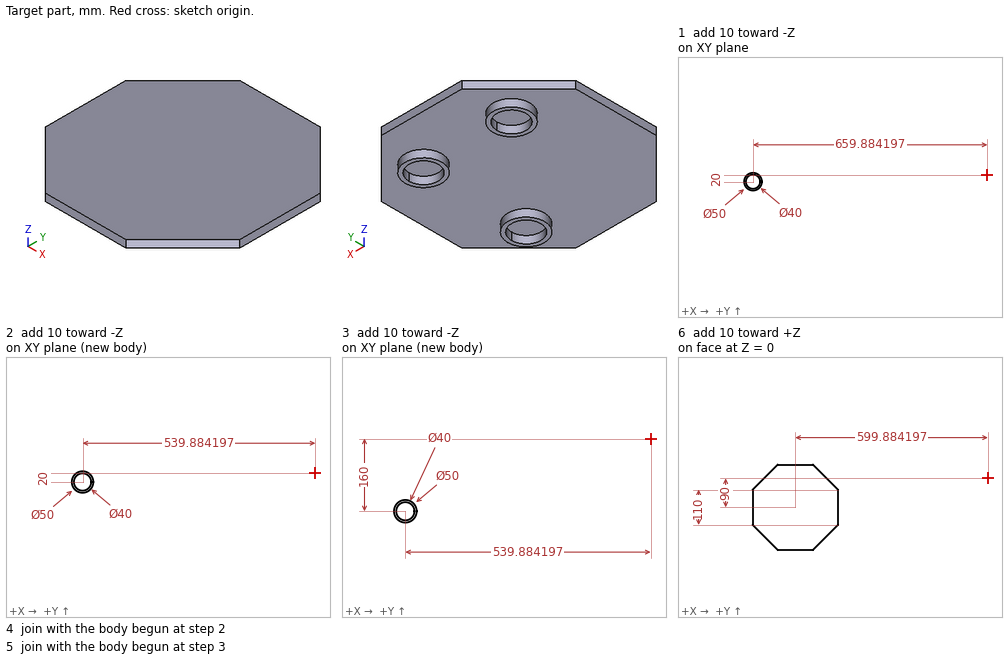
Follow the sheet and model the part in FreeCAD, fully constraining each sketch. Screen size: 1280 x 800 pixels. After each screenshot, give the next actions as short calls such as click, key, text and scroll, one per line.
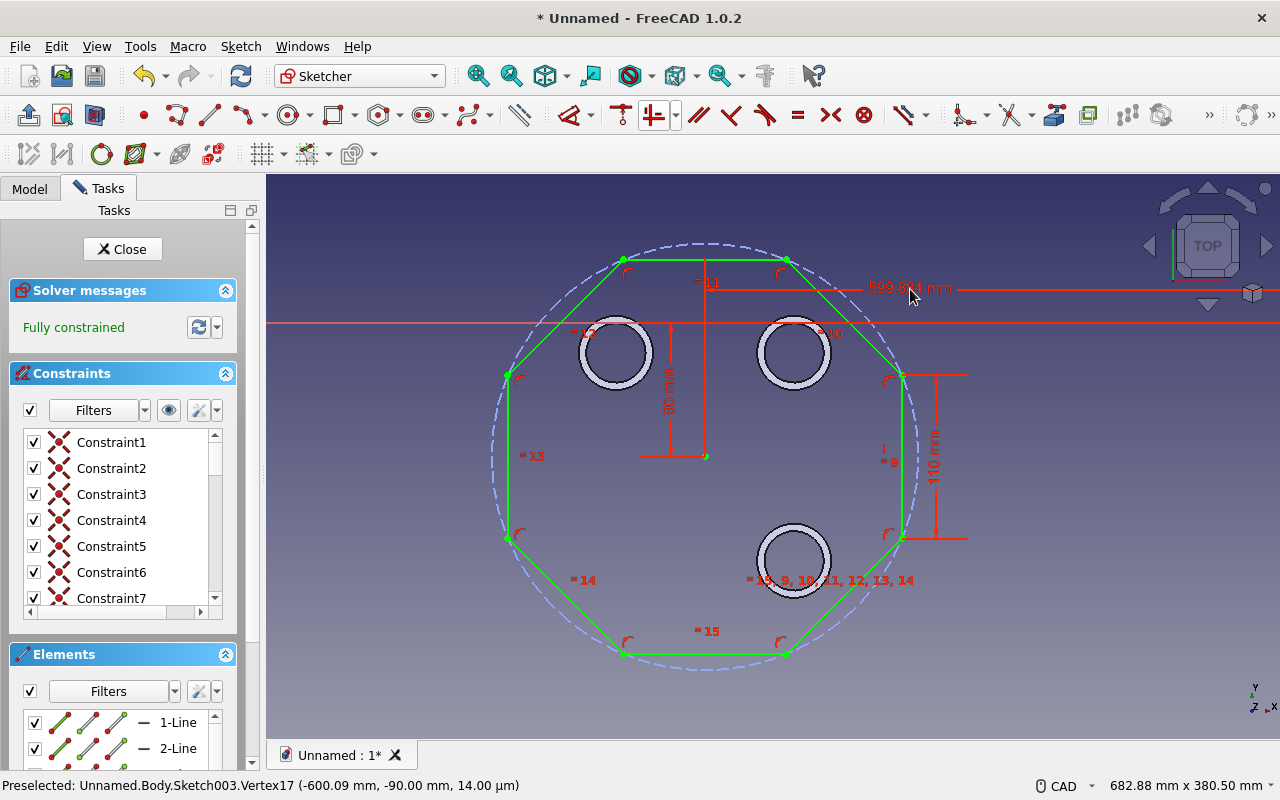
click(123, 249)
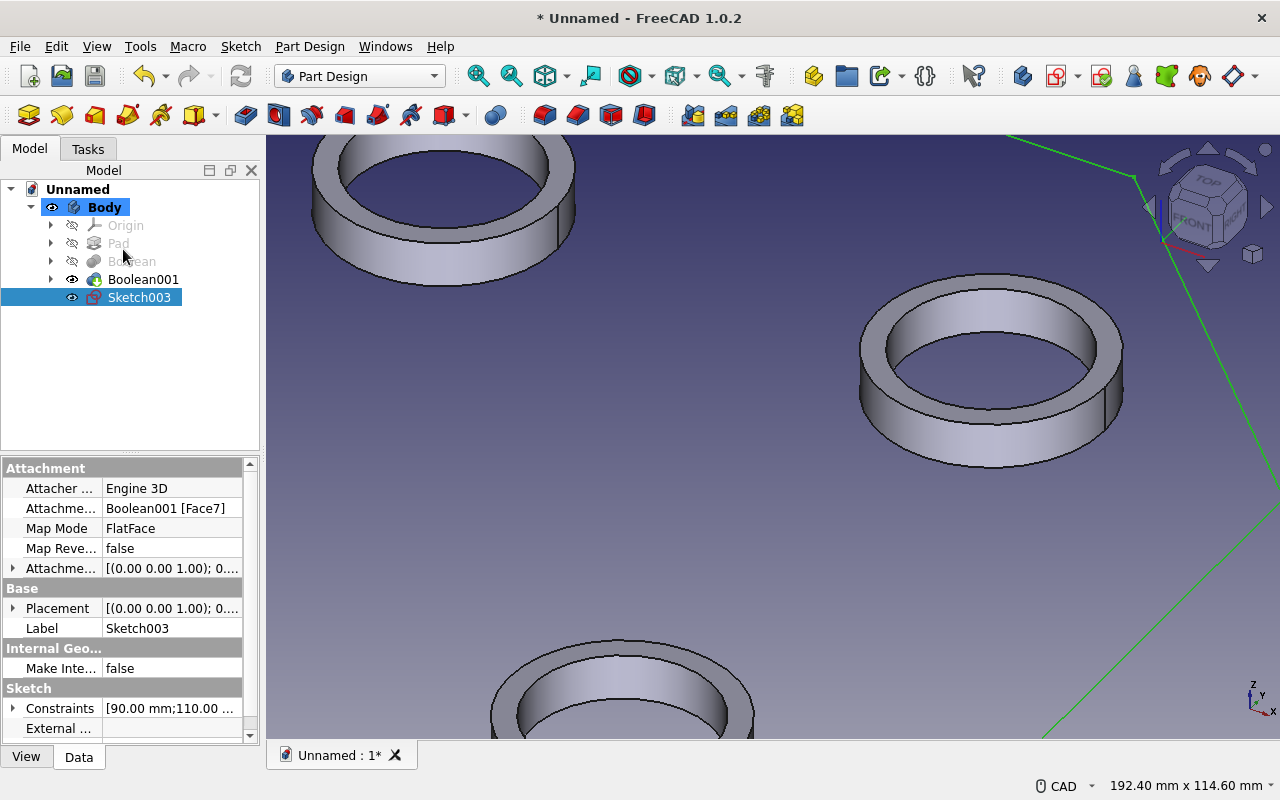
click(29, 116)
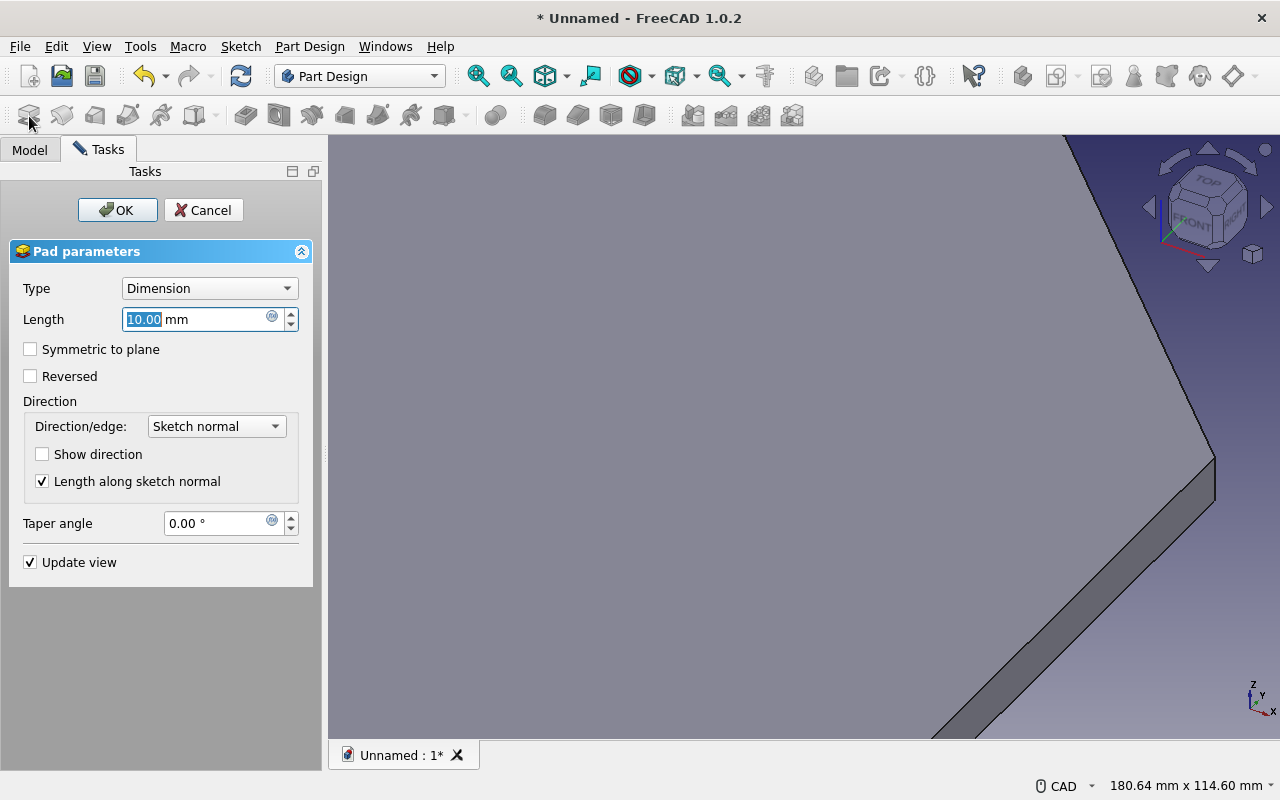
text(10)
key(Tab)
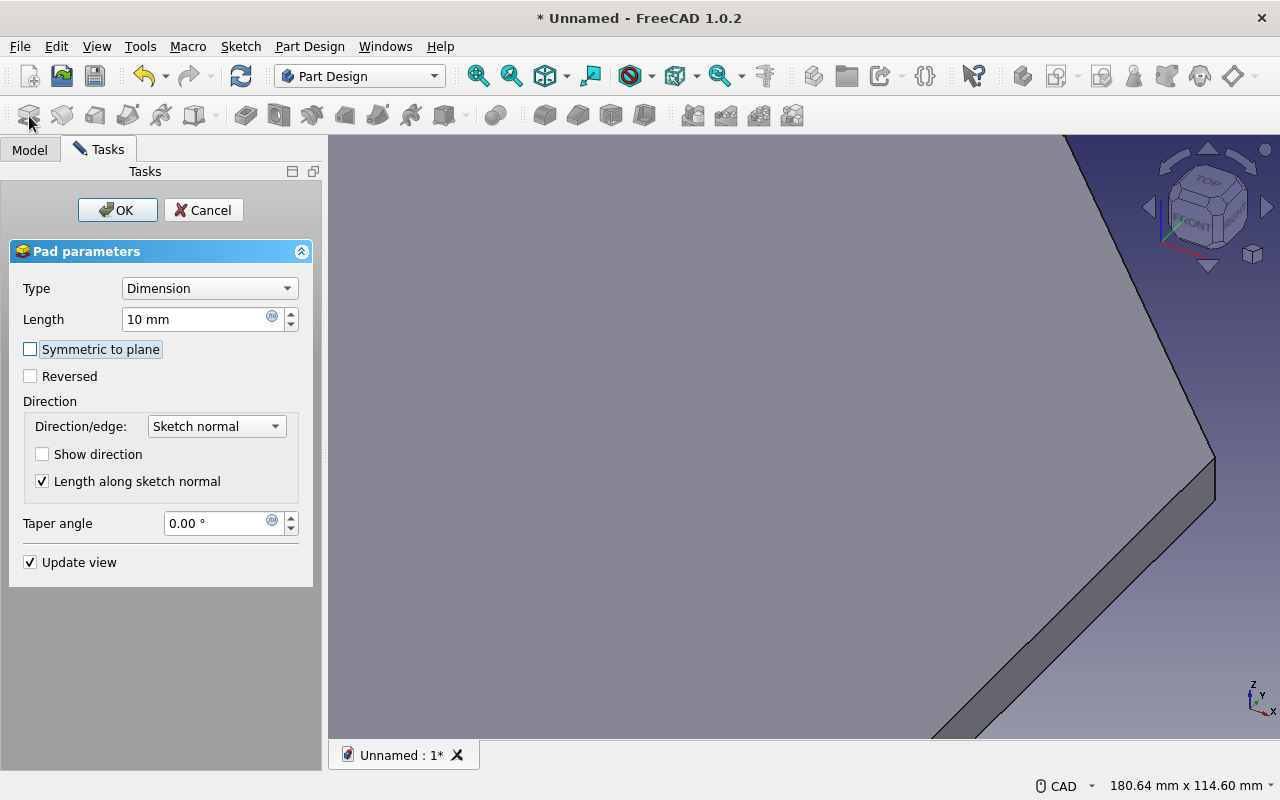
click(118, 210)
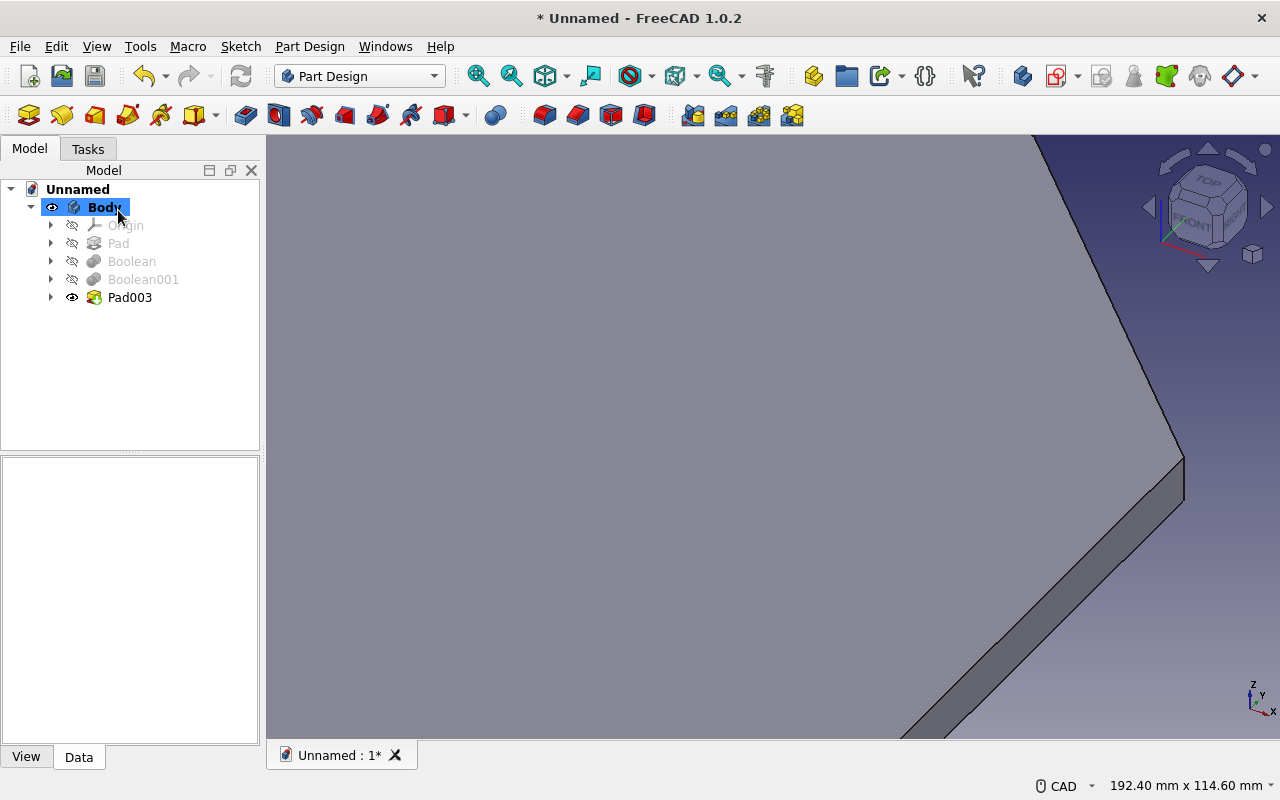
key(0)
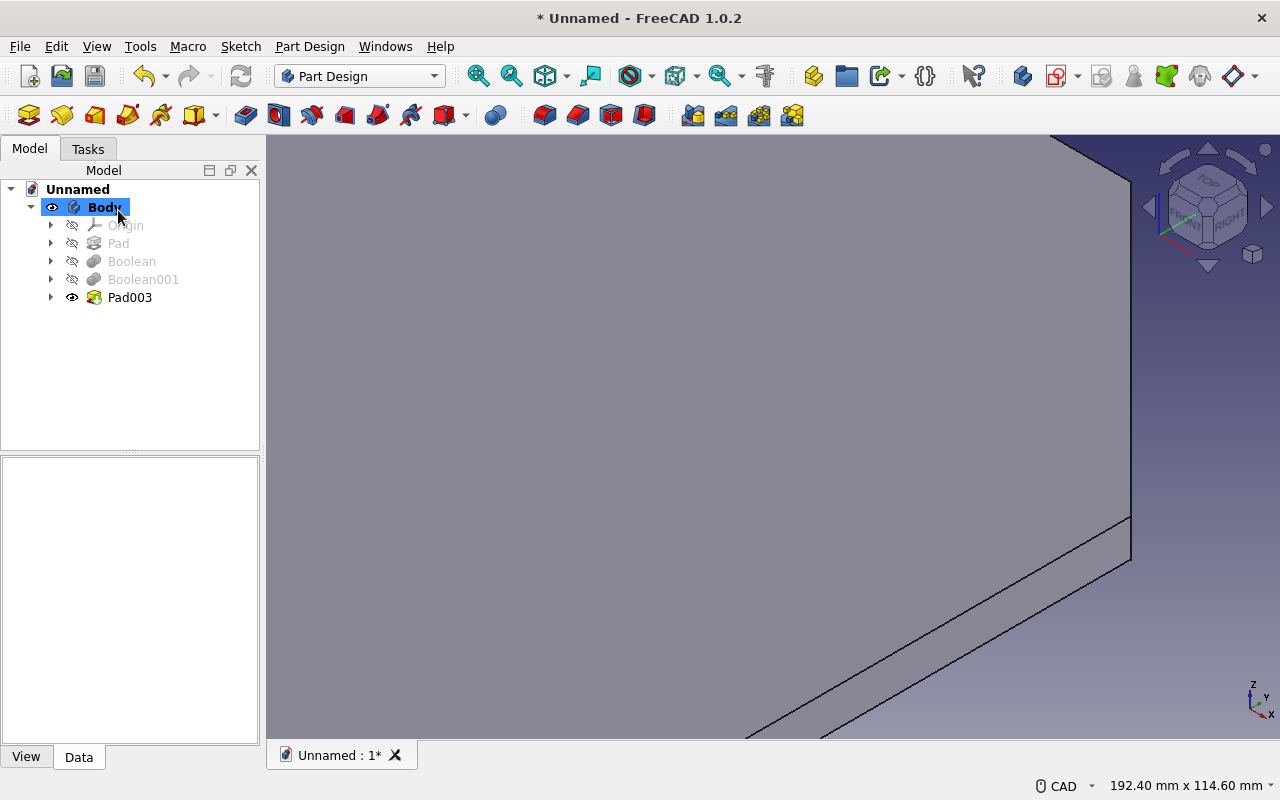
key(v)
key(f)